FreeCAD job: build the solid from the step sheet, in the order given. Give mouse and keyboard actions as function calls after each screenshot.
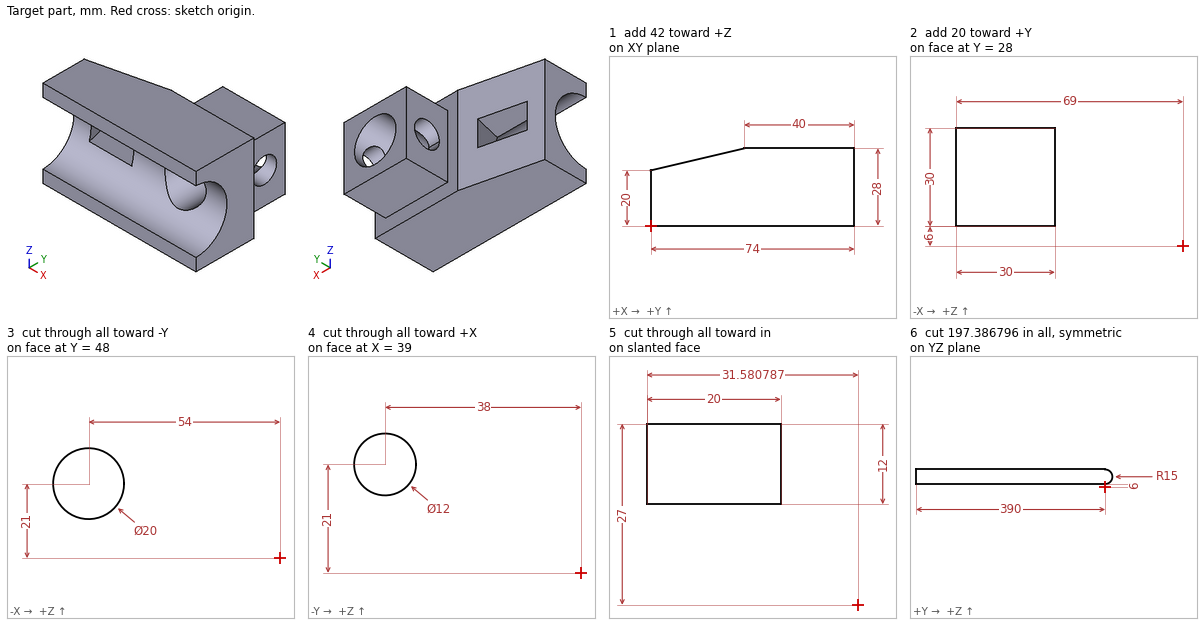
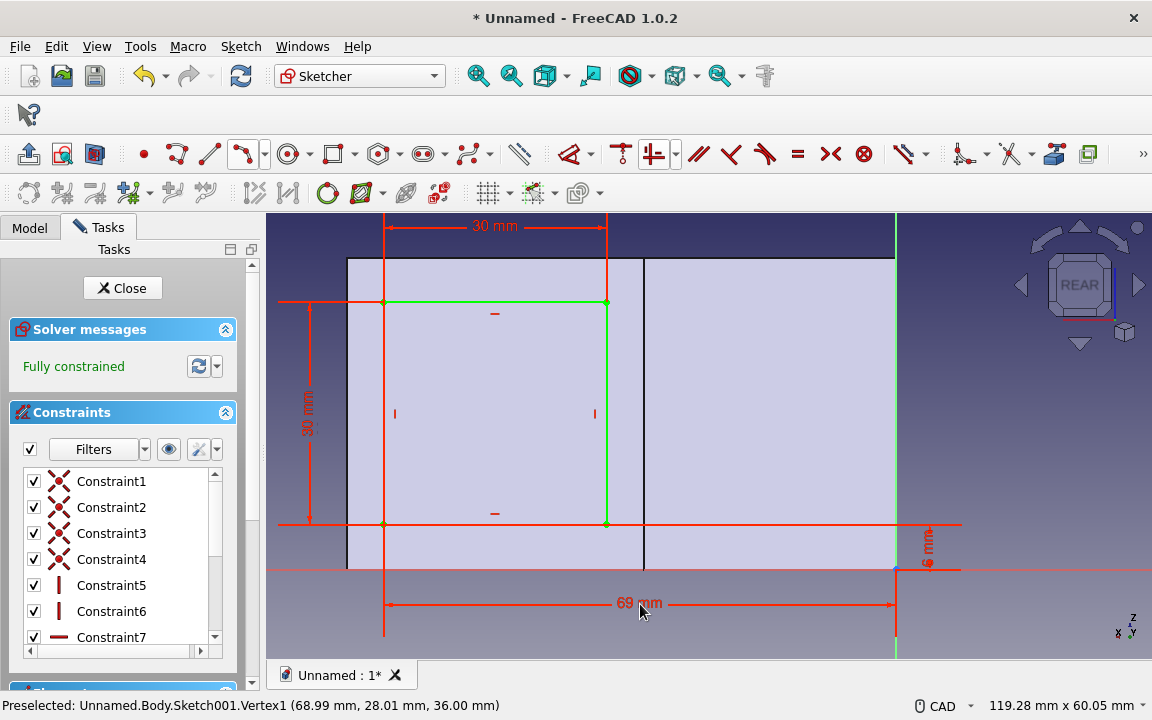
click(123, 288)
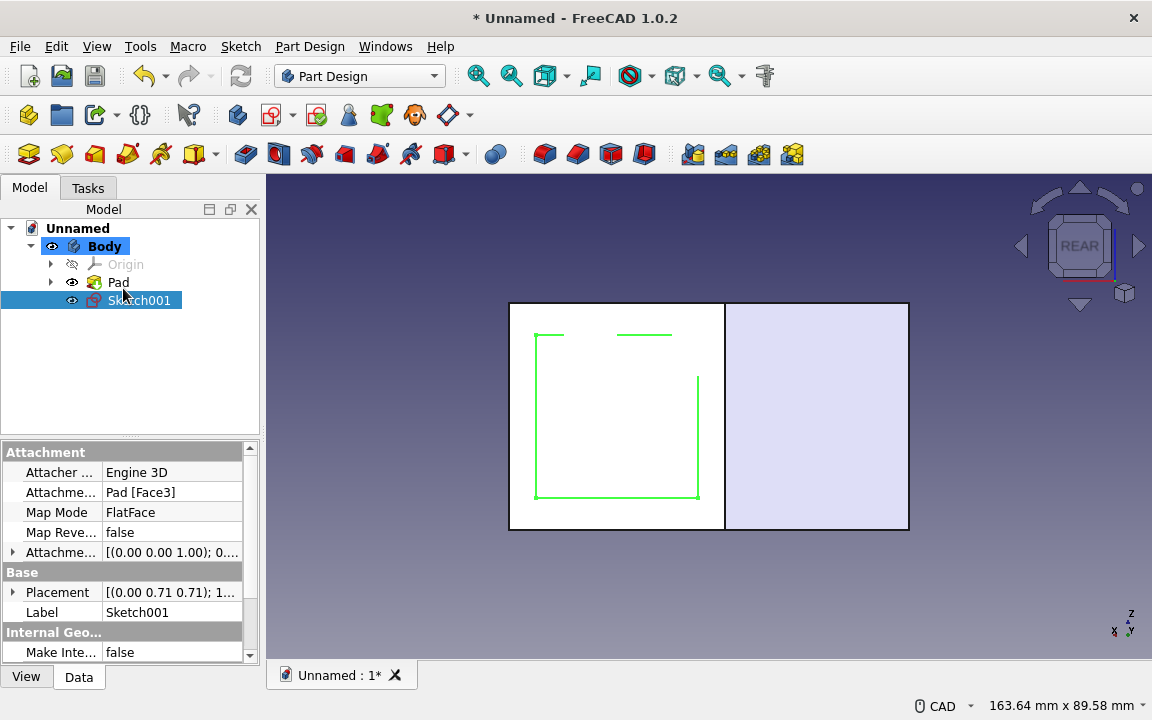
click(29, 154)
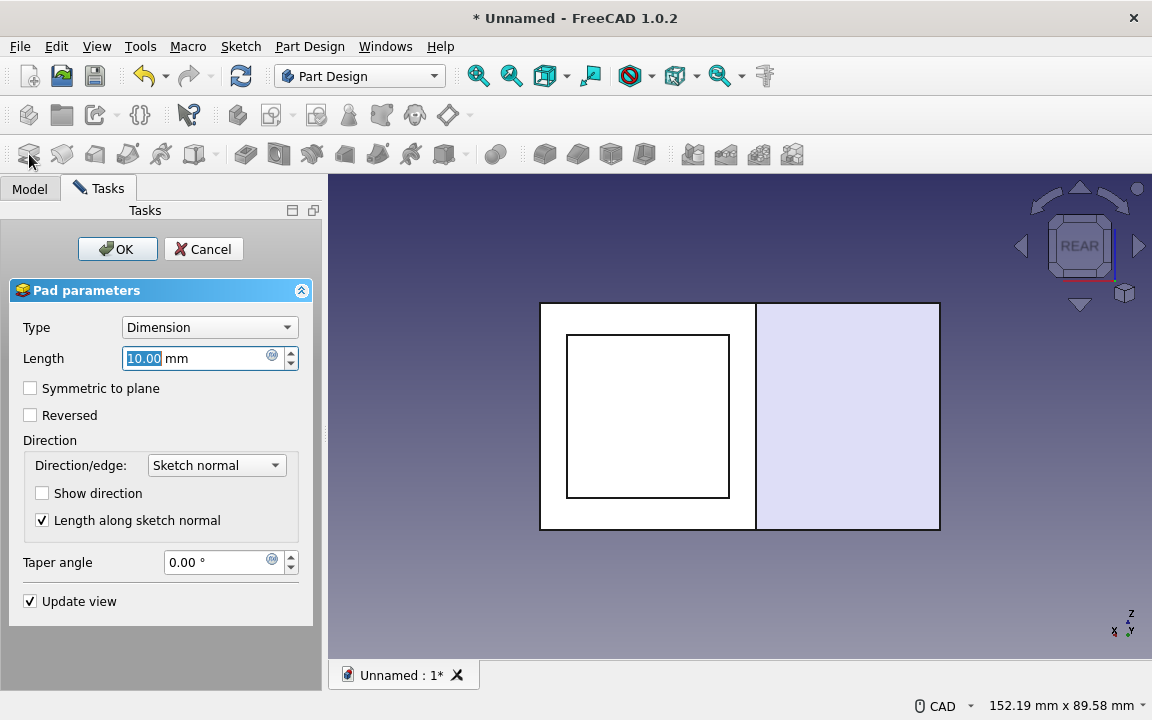
text(20)
key(Tab)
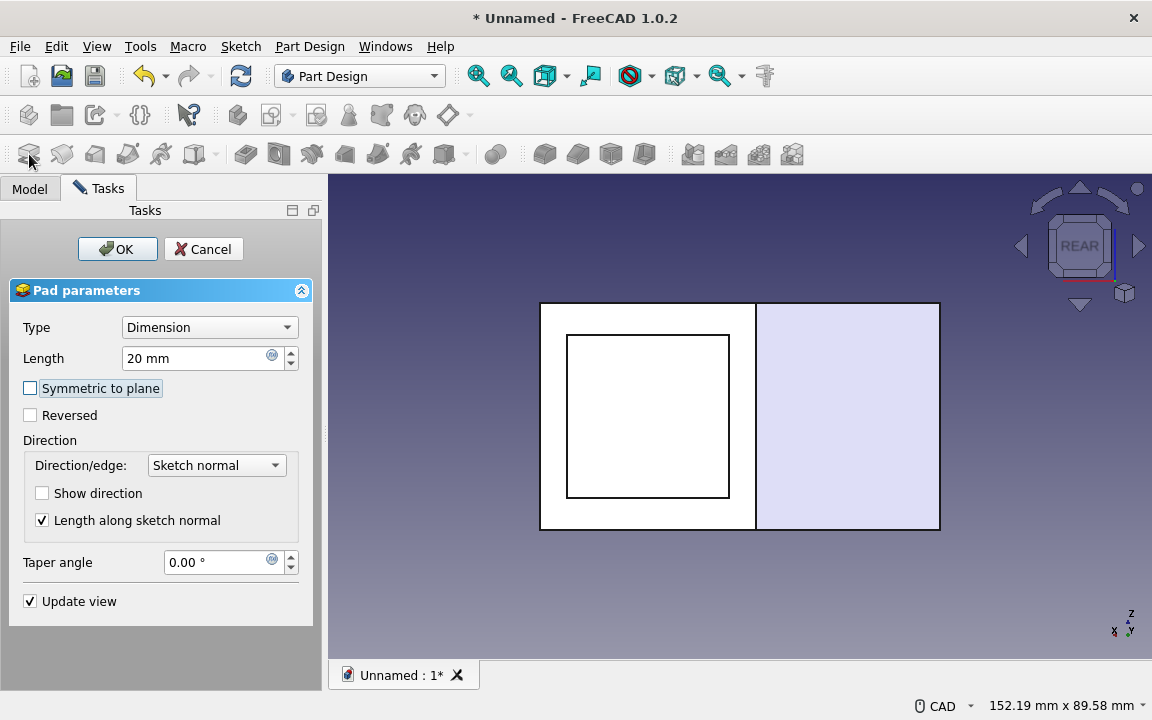
click(118, 249)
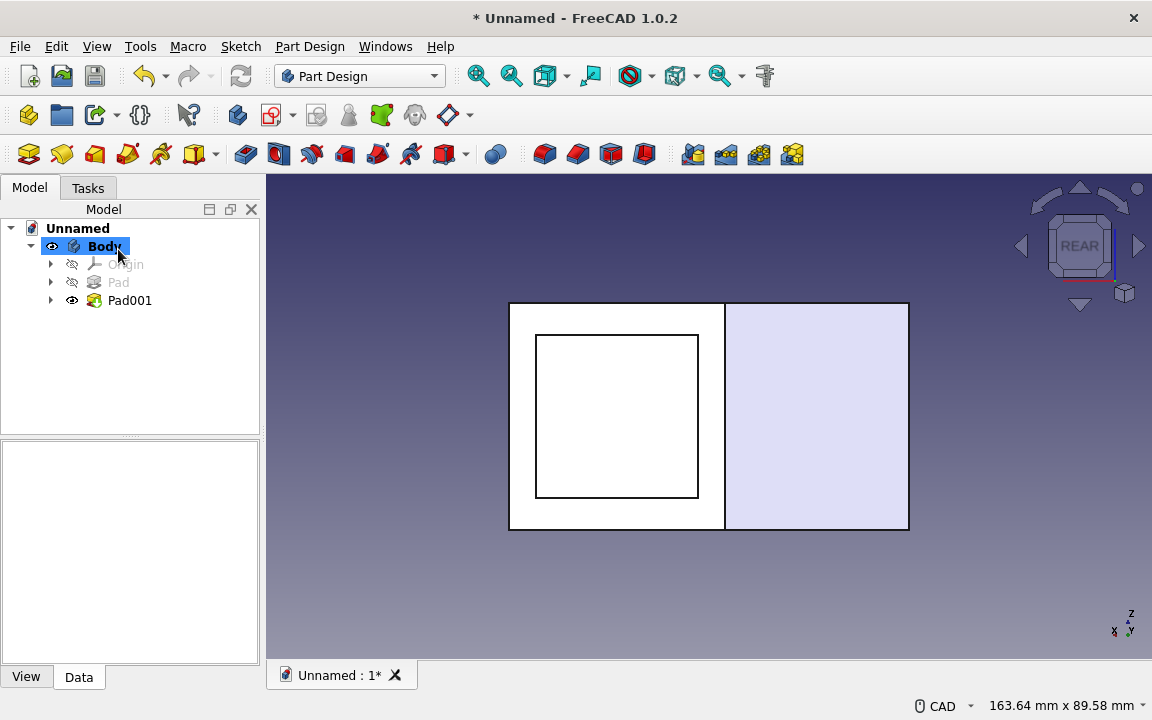
click(617, 415)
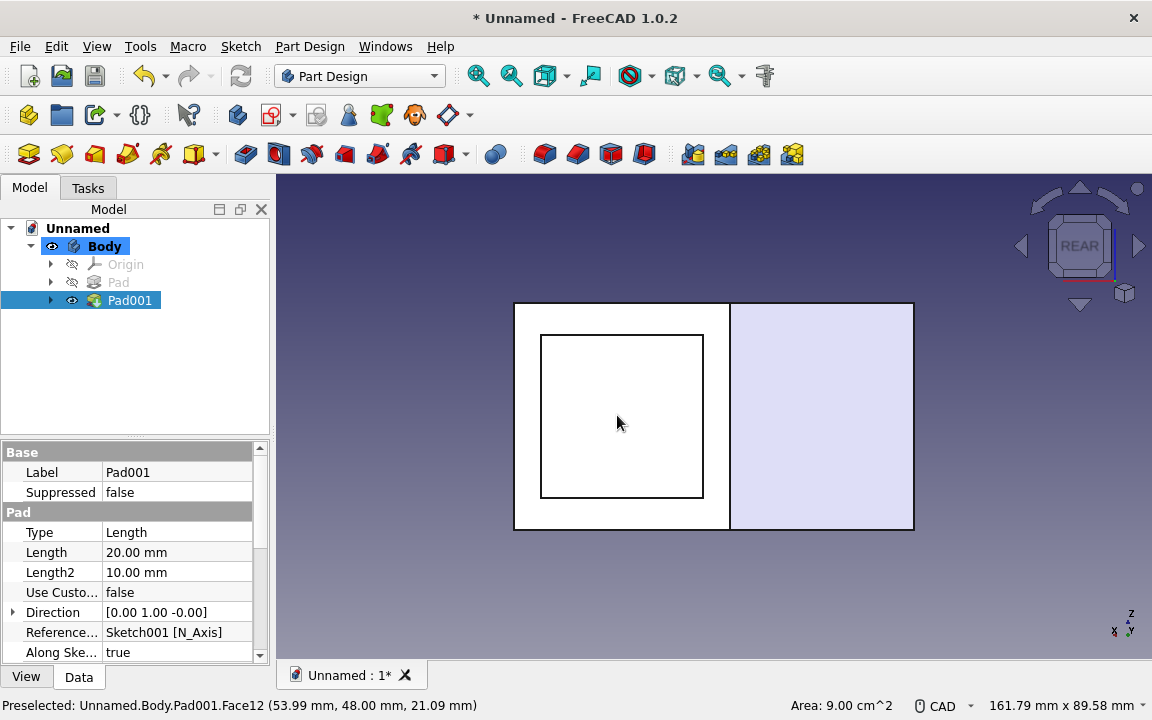
click(270, 116)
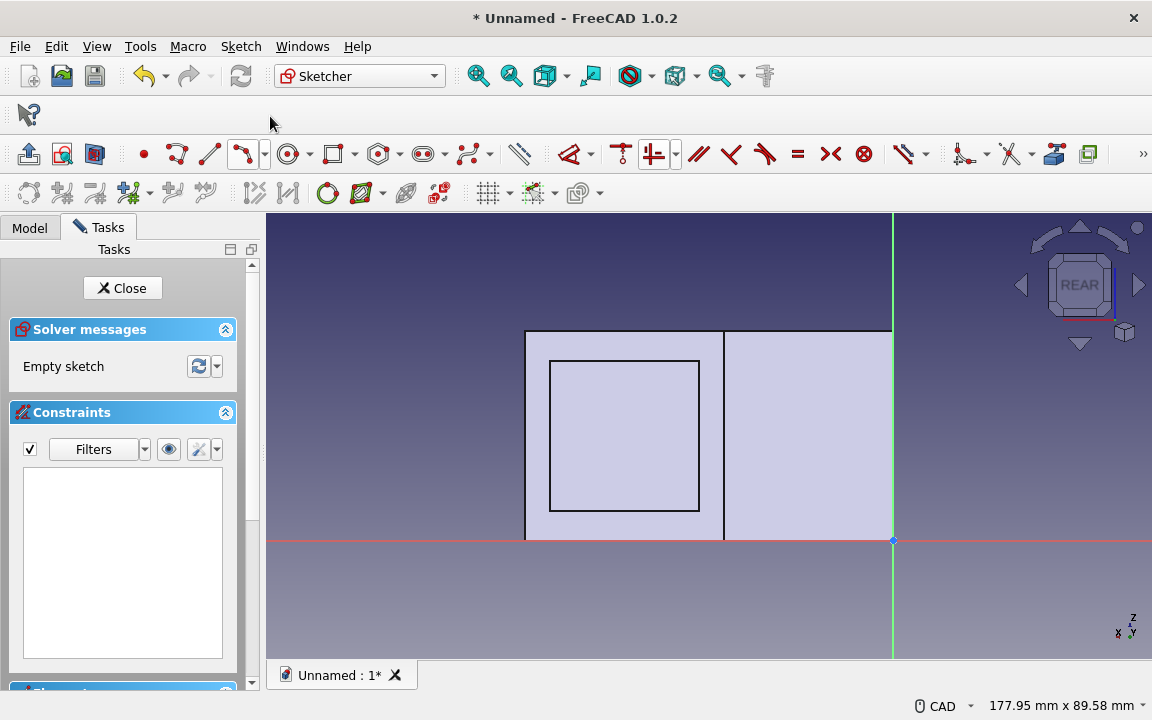
scroll(615, 436, up, 5)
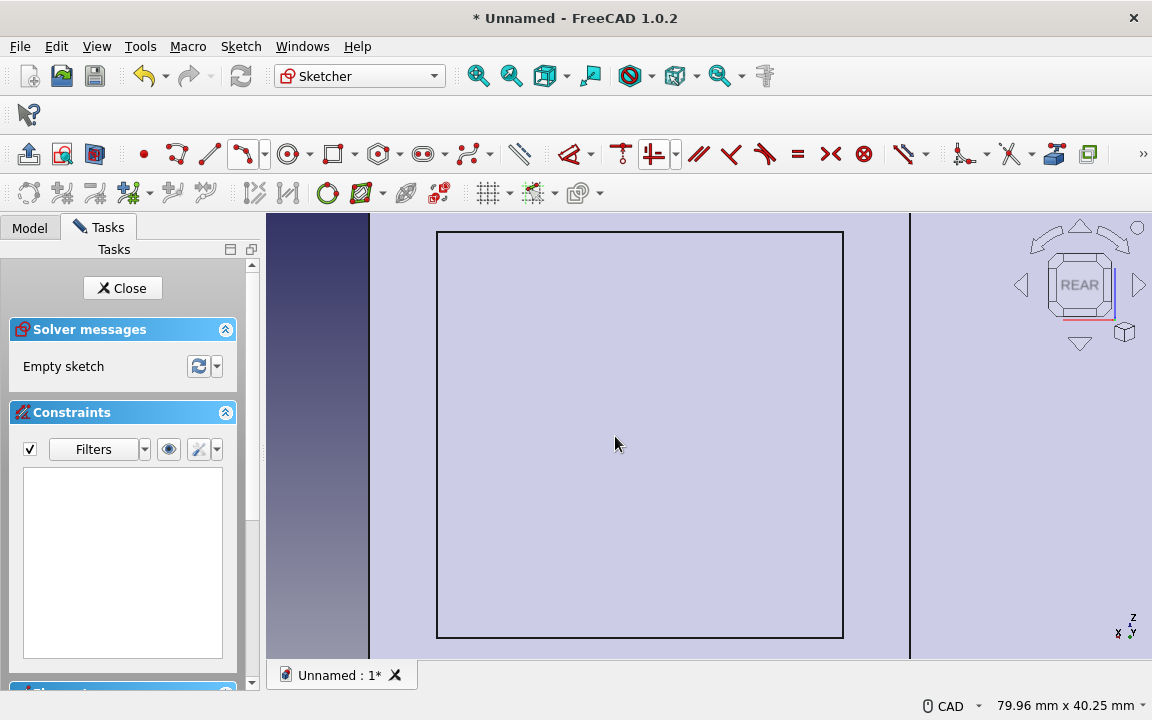
key(g)
key(c)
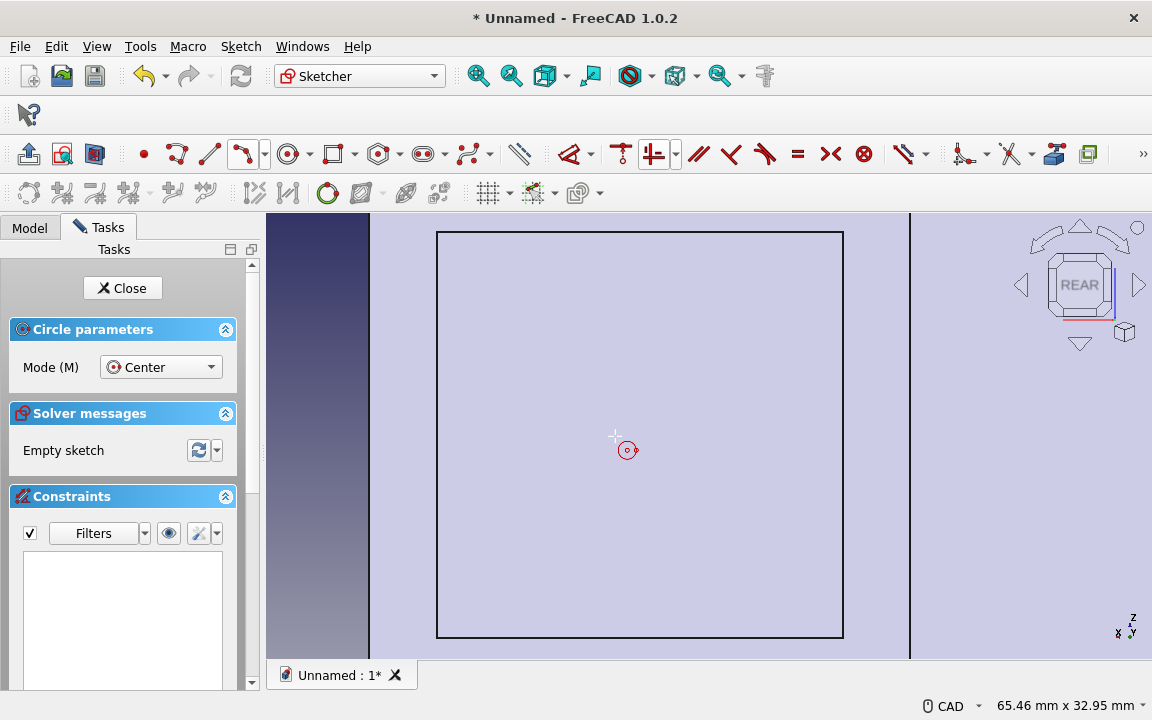
click(640, 435)
move(735, 339)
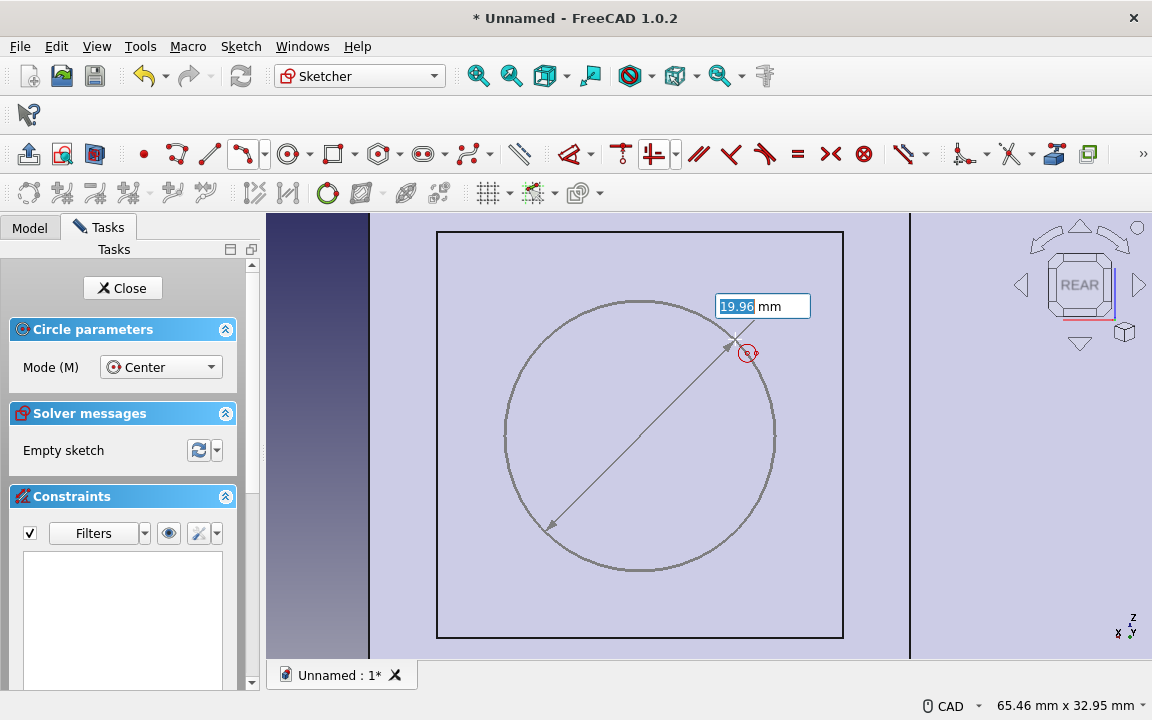
text(20)
key(Return)
key(Escape)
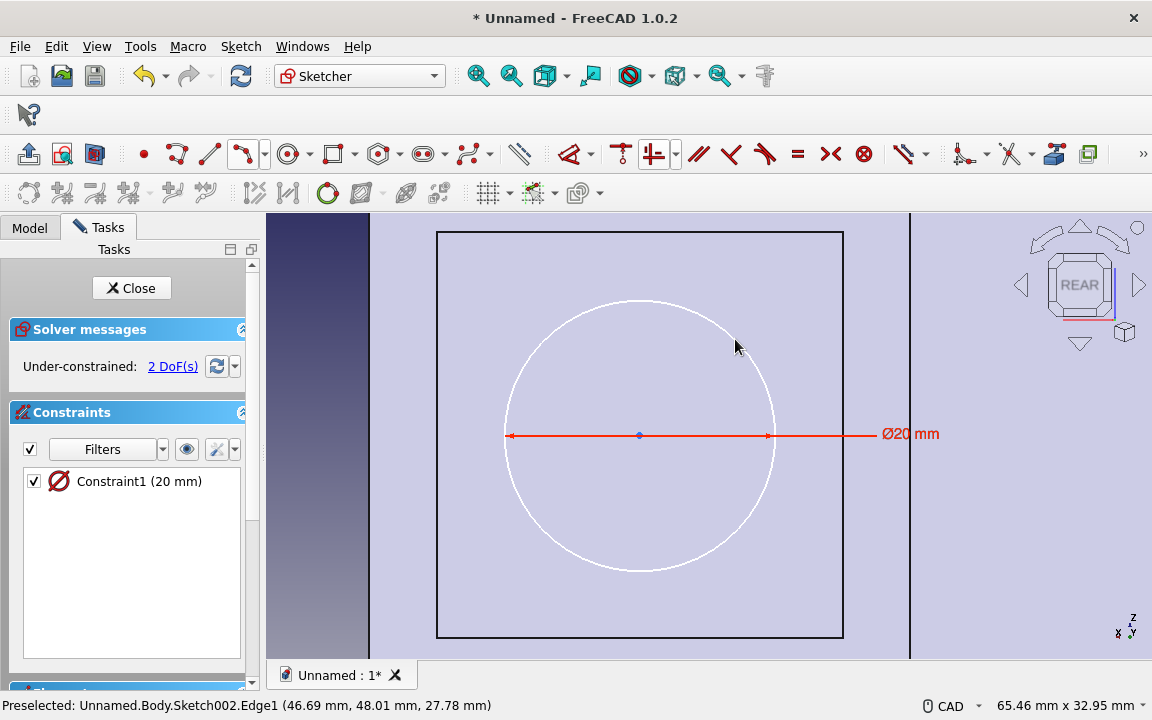
click(568, 154)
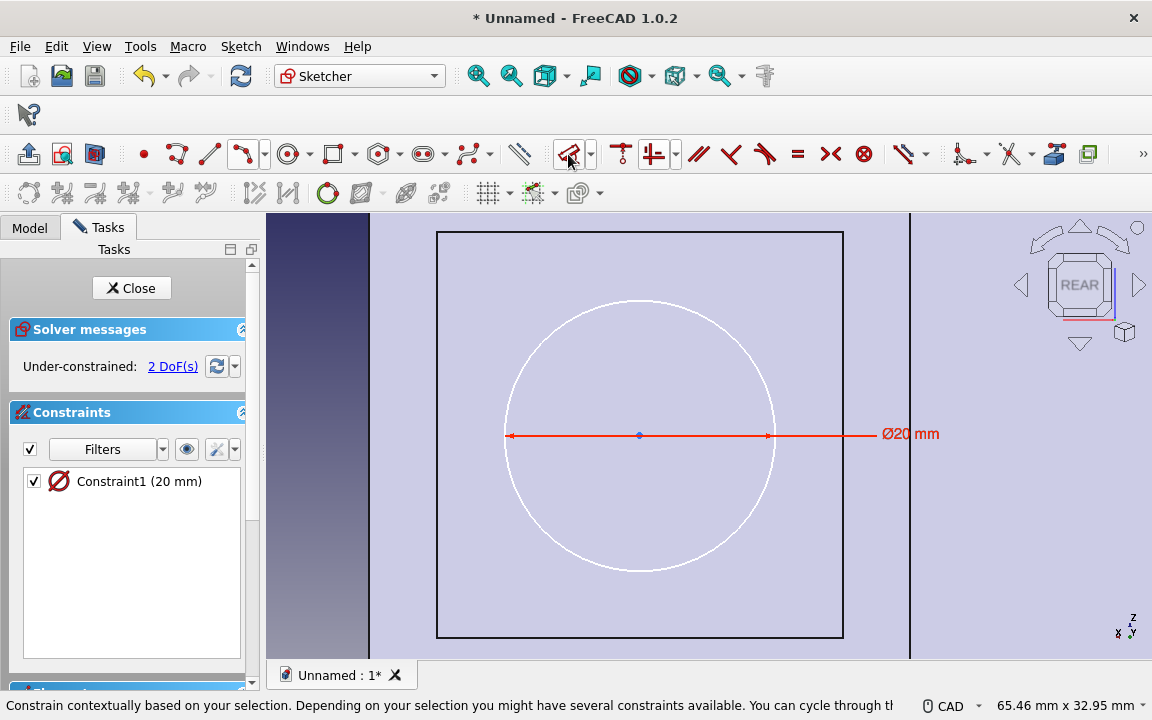
click(640, 436)
click(813, 402)